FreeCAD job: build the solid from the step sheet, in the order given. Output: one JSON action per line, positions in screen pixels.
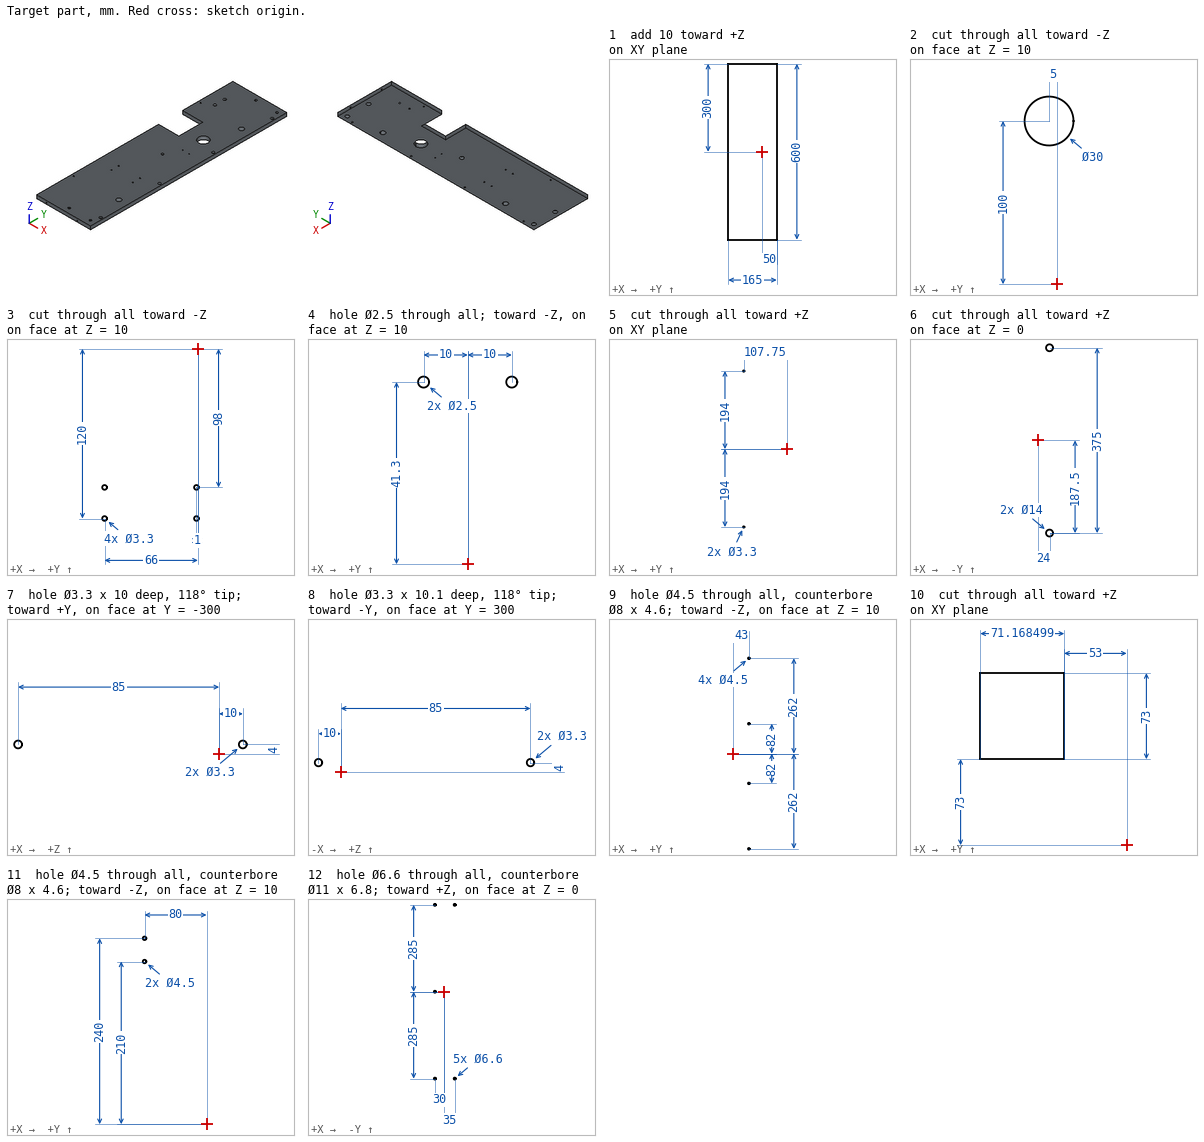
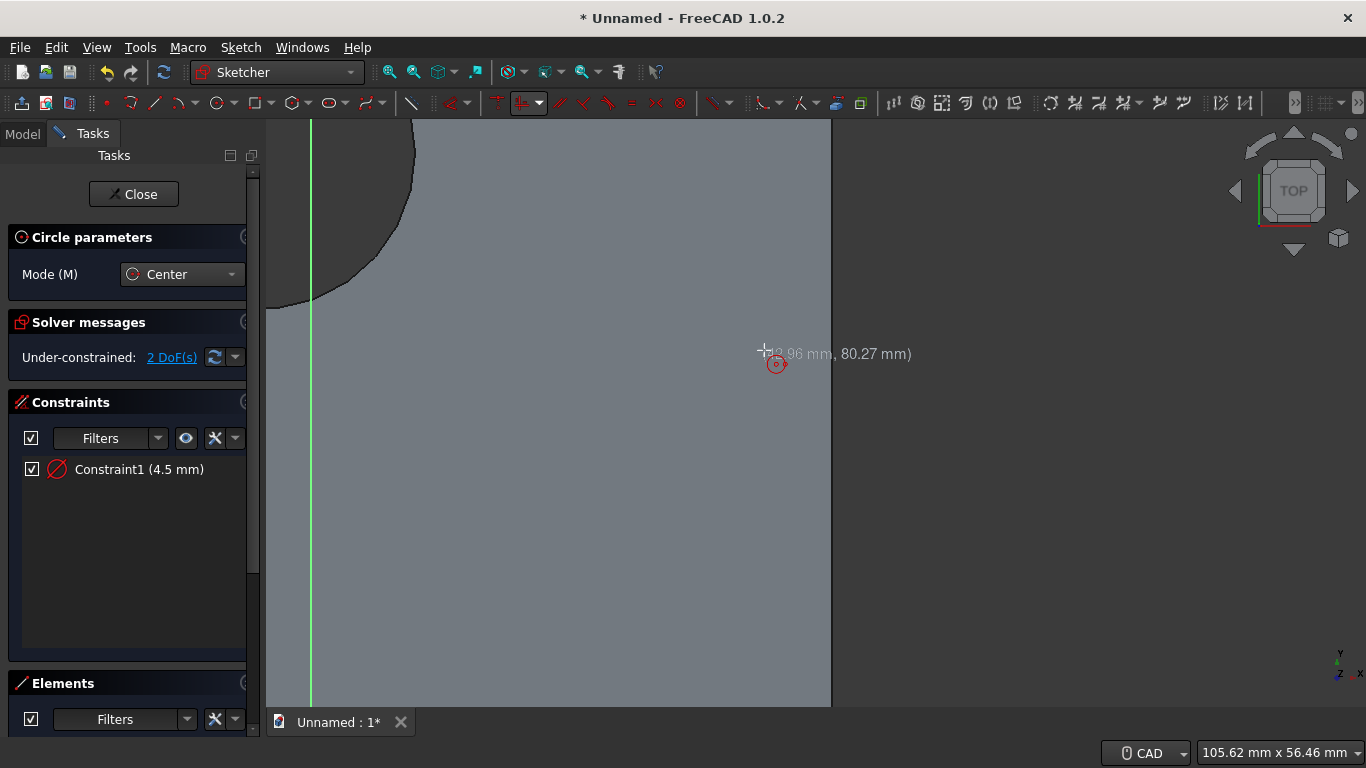
{"action": "scroll", "coordinate": [764, 350], "scroll_direction": "down", "scroll_amount": 13}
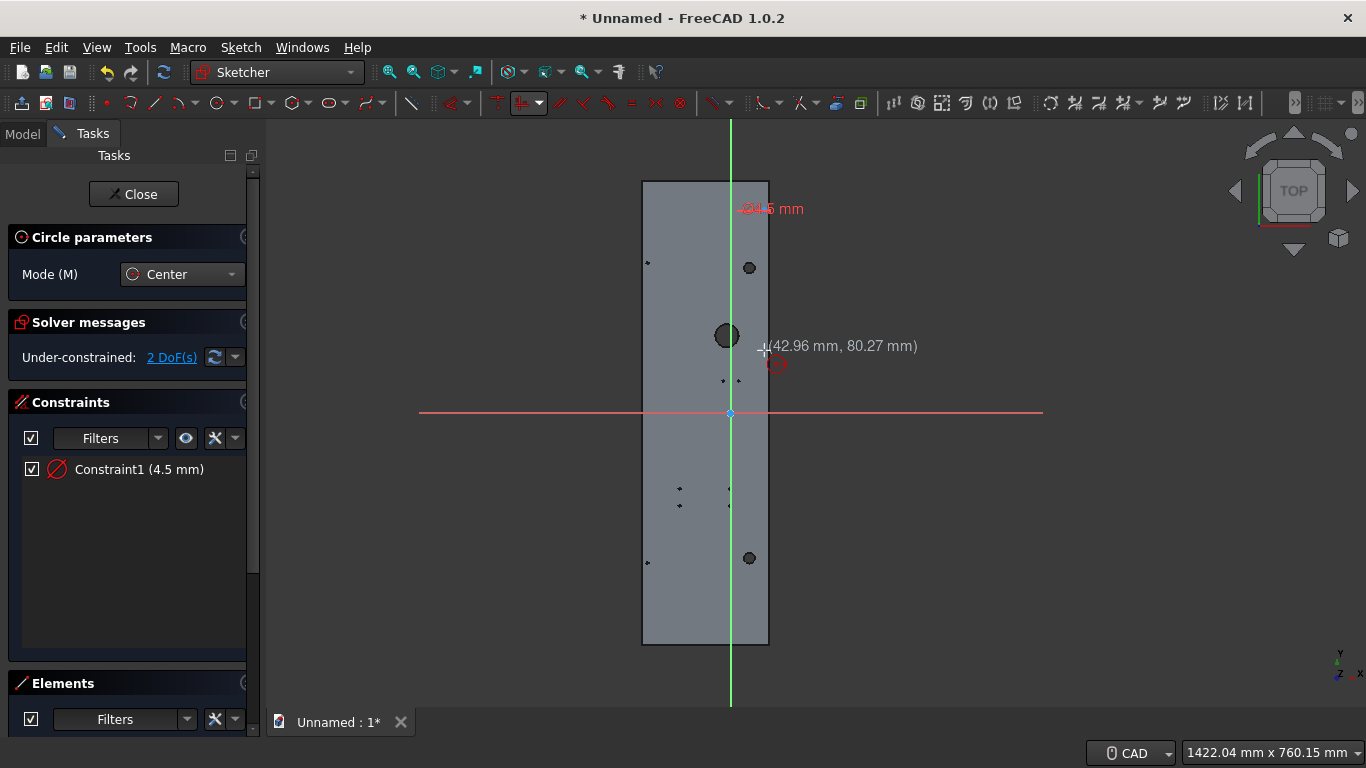
{"action": "left_click", "coordinate": [764, 350]}
{"action": "mouse_move", "coordinate": [765, 348]}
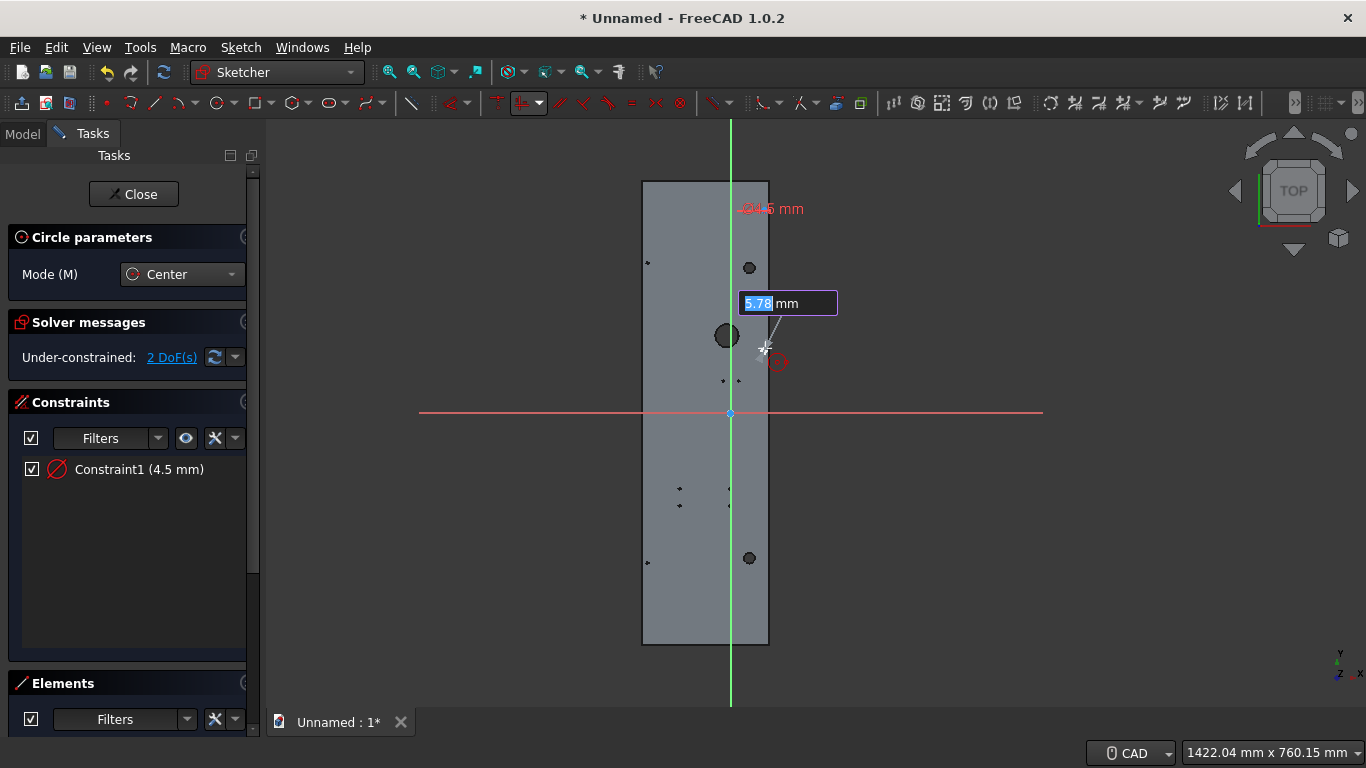
{"action": "type", "text": "4.5"}
{"action": "key", "text": "Return"}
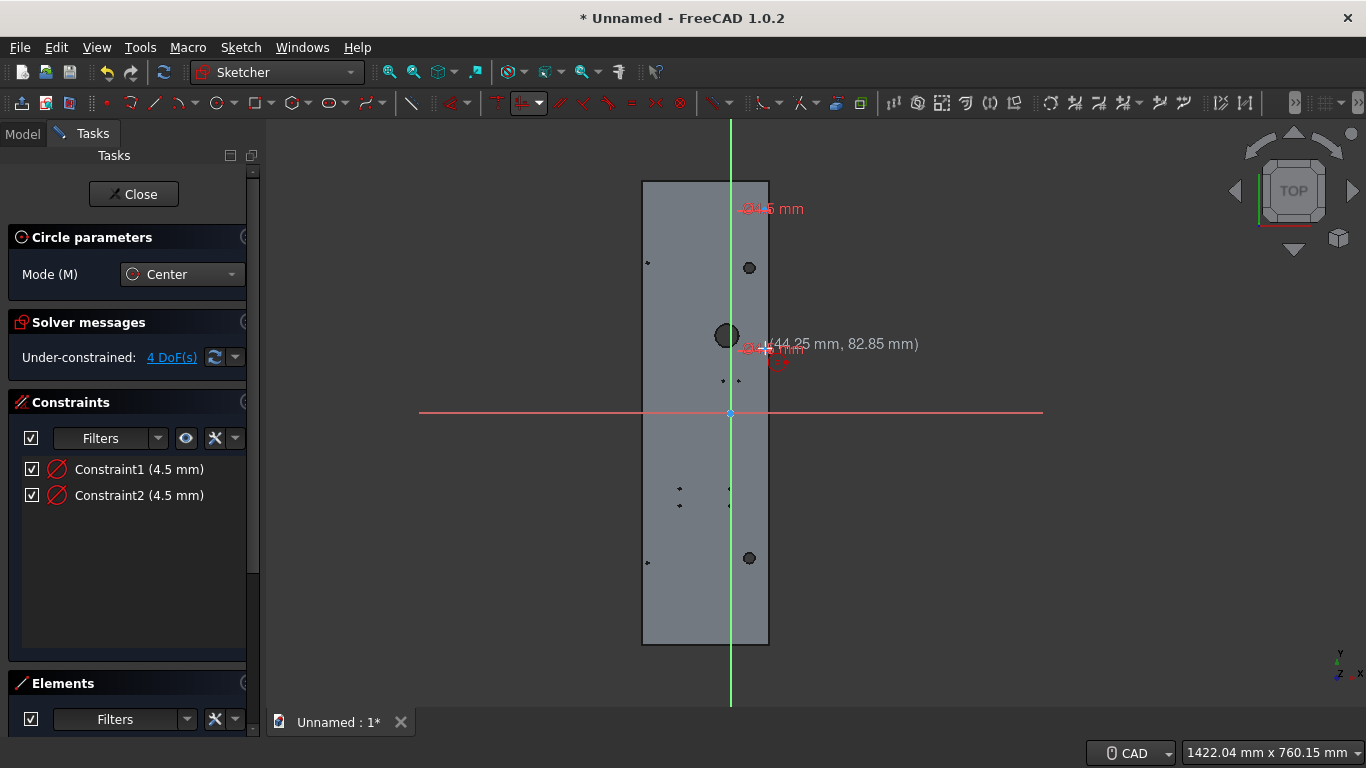
{"action": "scroll", "coordinate": [764, 477], "scroll_direction": "up", "scroll_amount": 13}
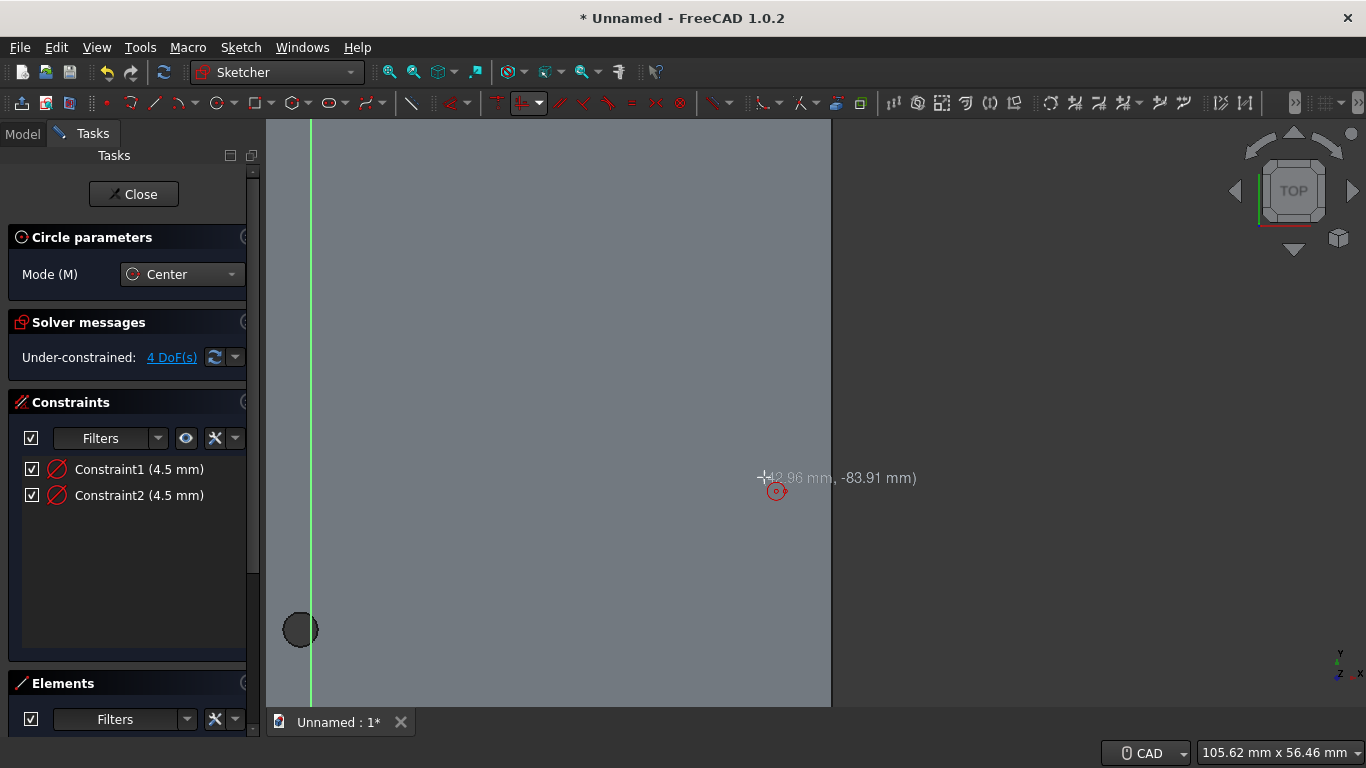
{"action": "scroll", "coordinate": [764, 478], "scroll_direction": "down", "scroll_amount": 13}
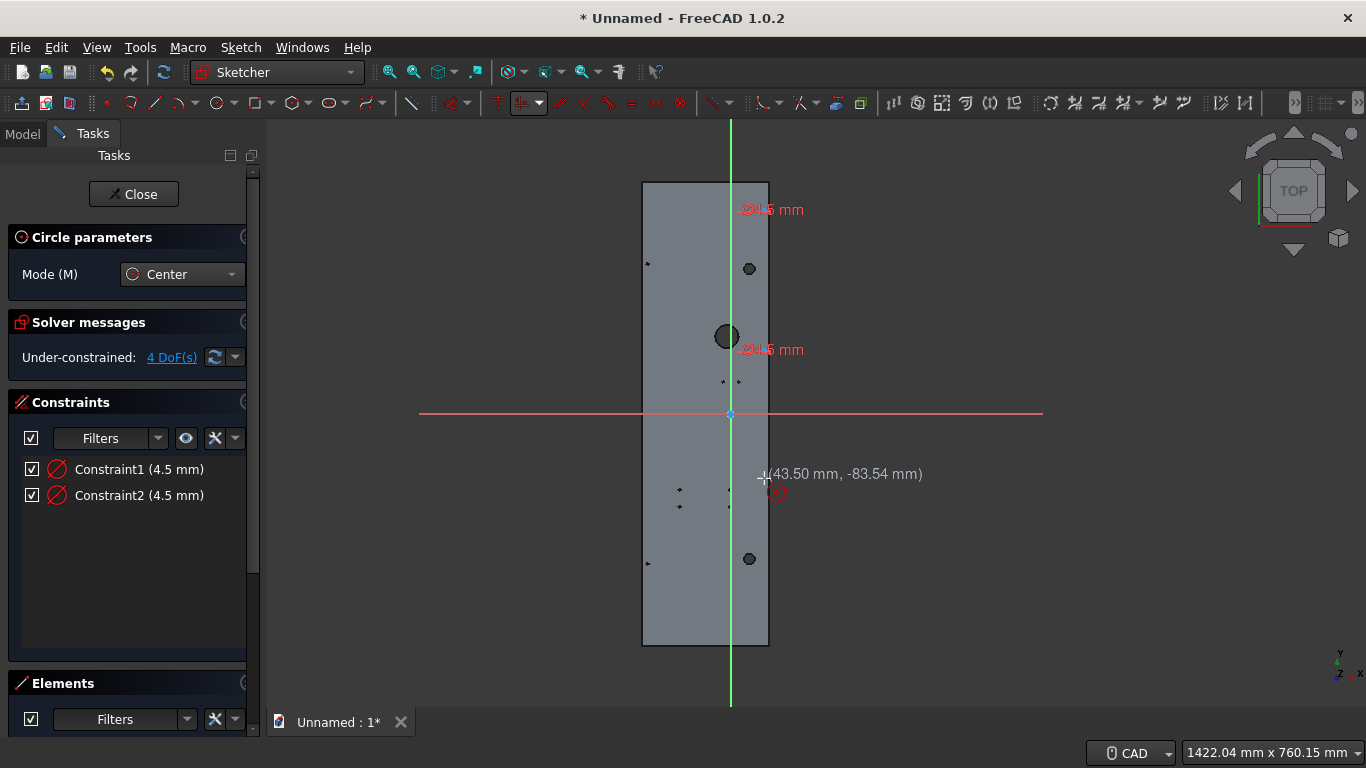
{"action": "left_click", "coordinate": [764, 477]}
{"action": "mouse_move", "coordinate": [765, 476]}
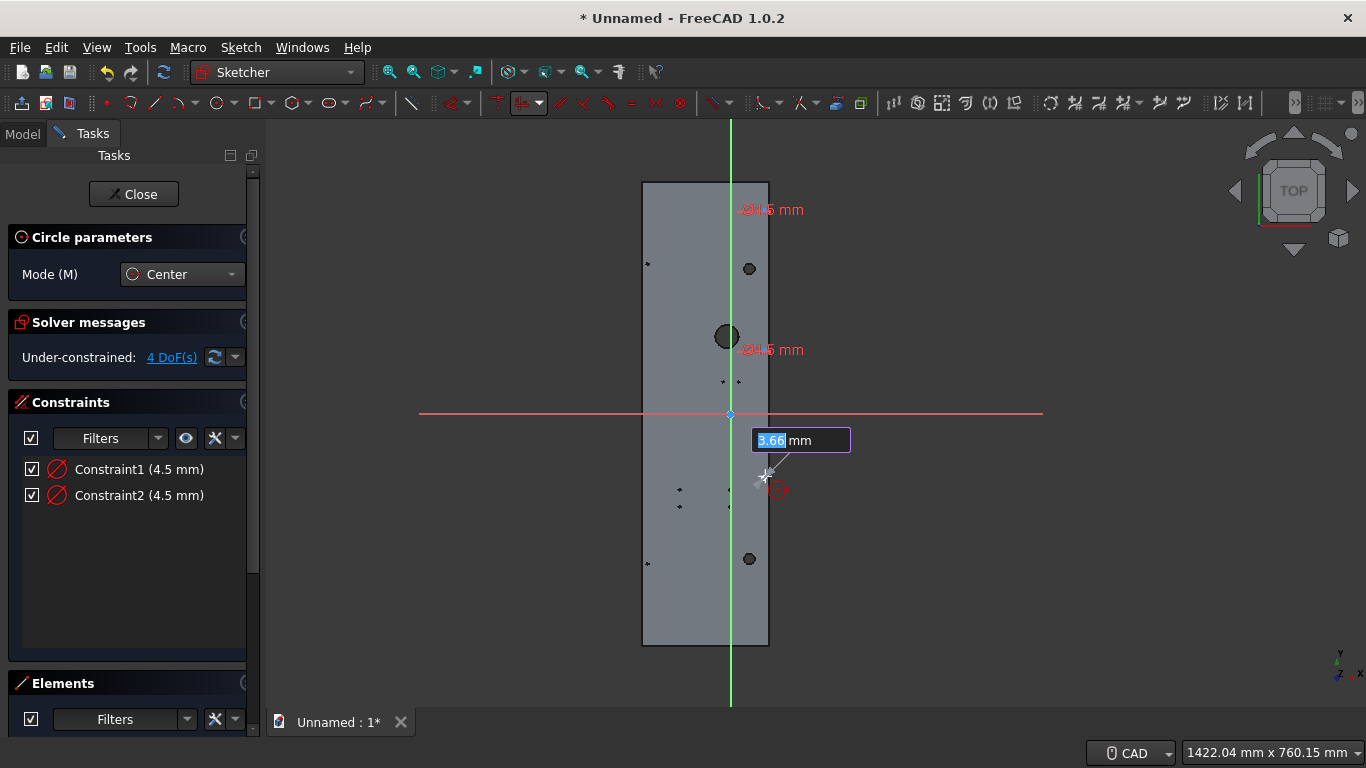
{"action": "type", "text": "4.5"}
{"action": "key", "text": "Return"}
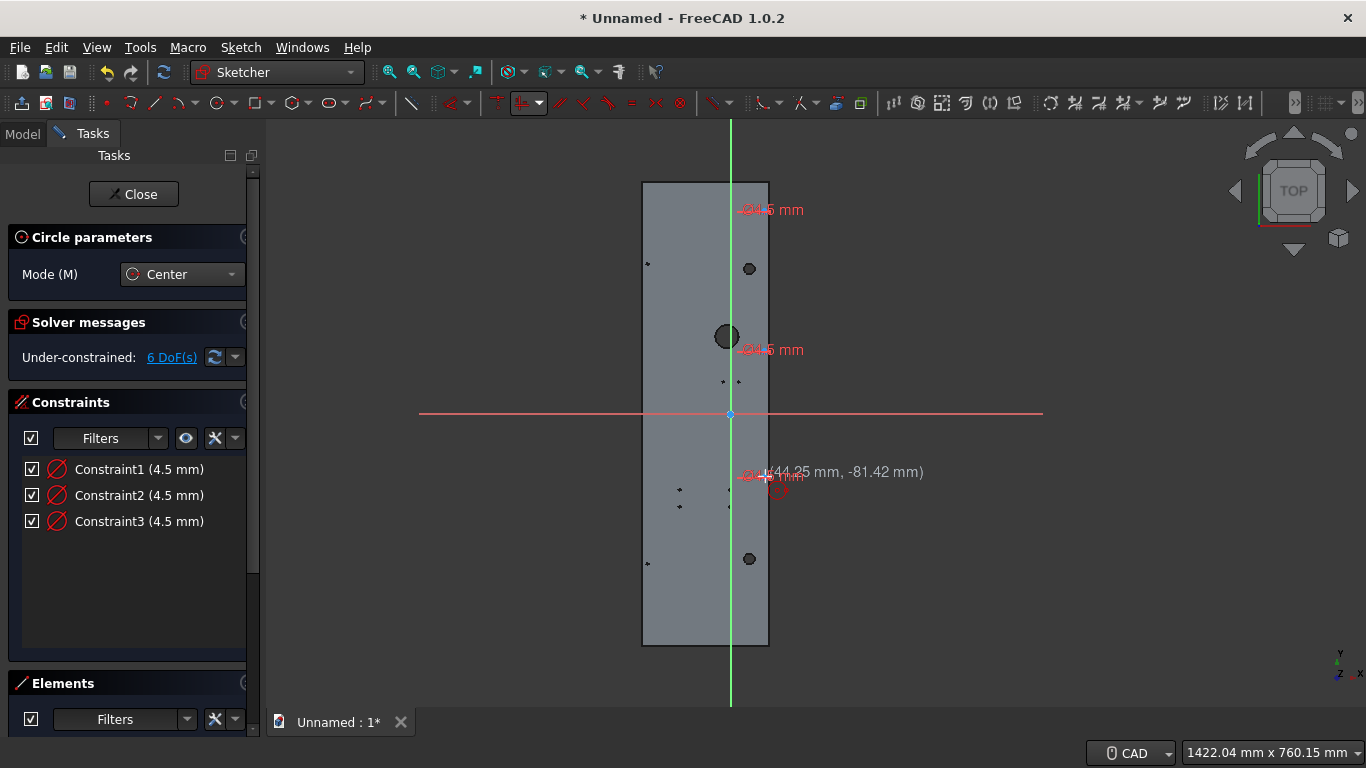
{"action": "scroll", "coordinate": [764, 617], "scroll_direction": "up", "scroll_amount": 13}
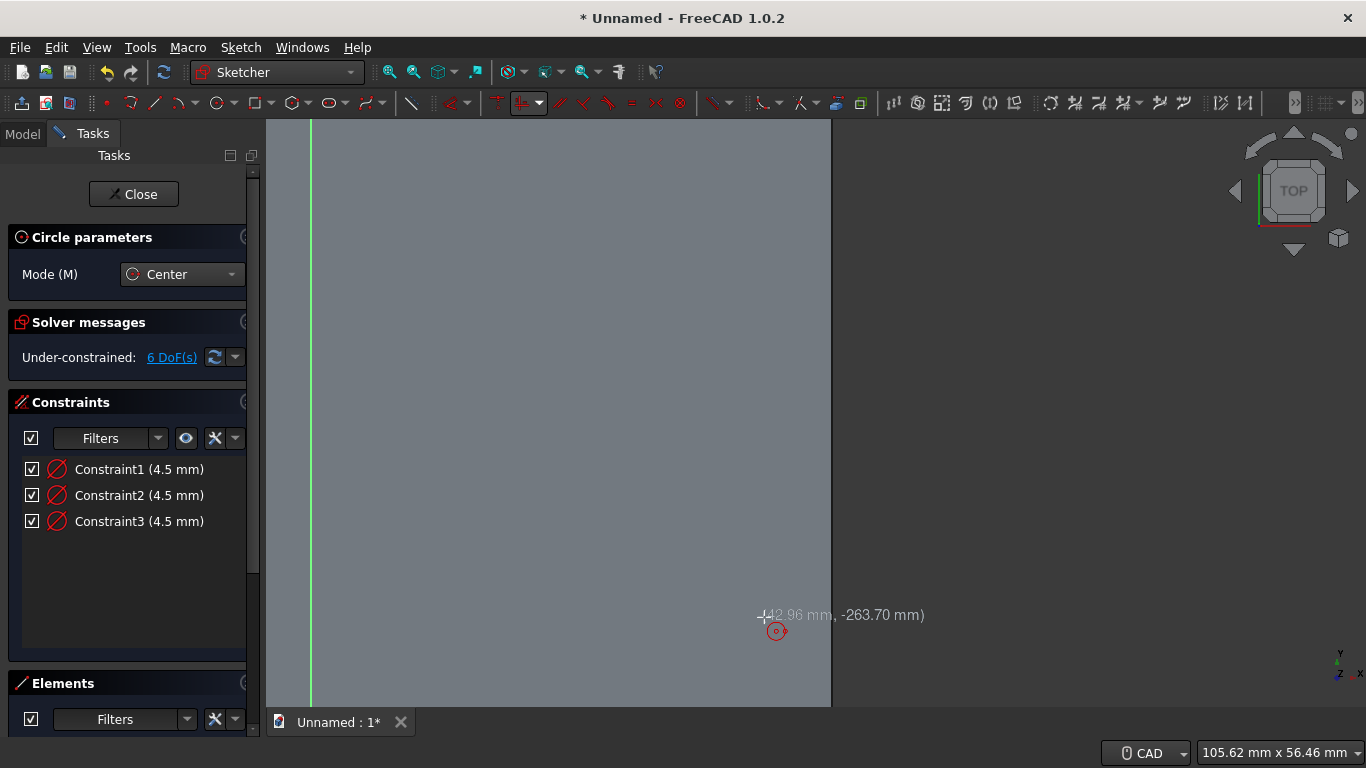
{"action": "scroll", "coordinate": [764, 617], "scroll_direction": "down", "scroll_amount": 13}